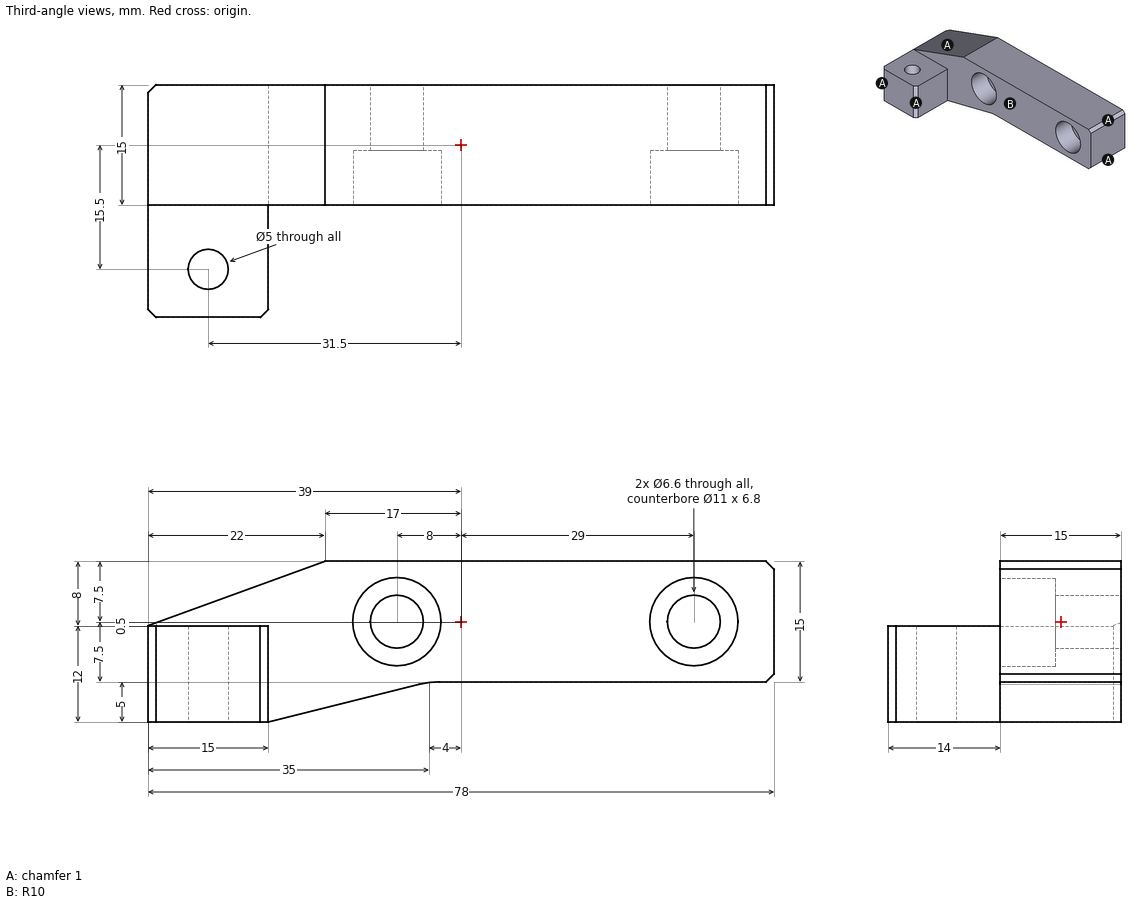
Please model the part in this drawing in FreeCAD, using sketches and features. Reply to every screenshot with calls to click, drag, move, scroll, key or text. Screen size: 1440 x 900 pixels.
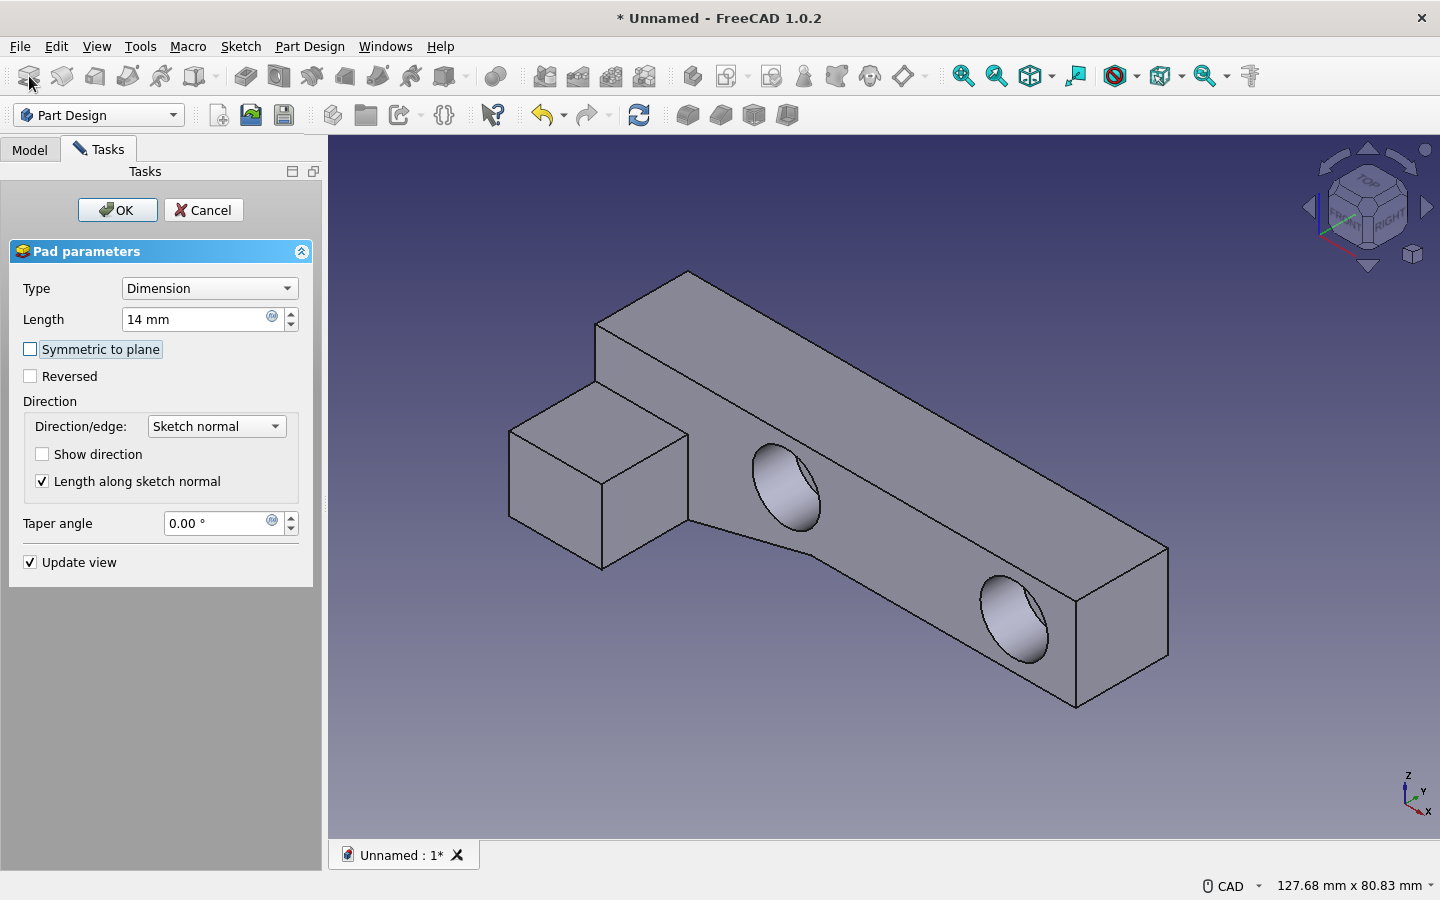
click(118, 210)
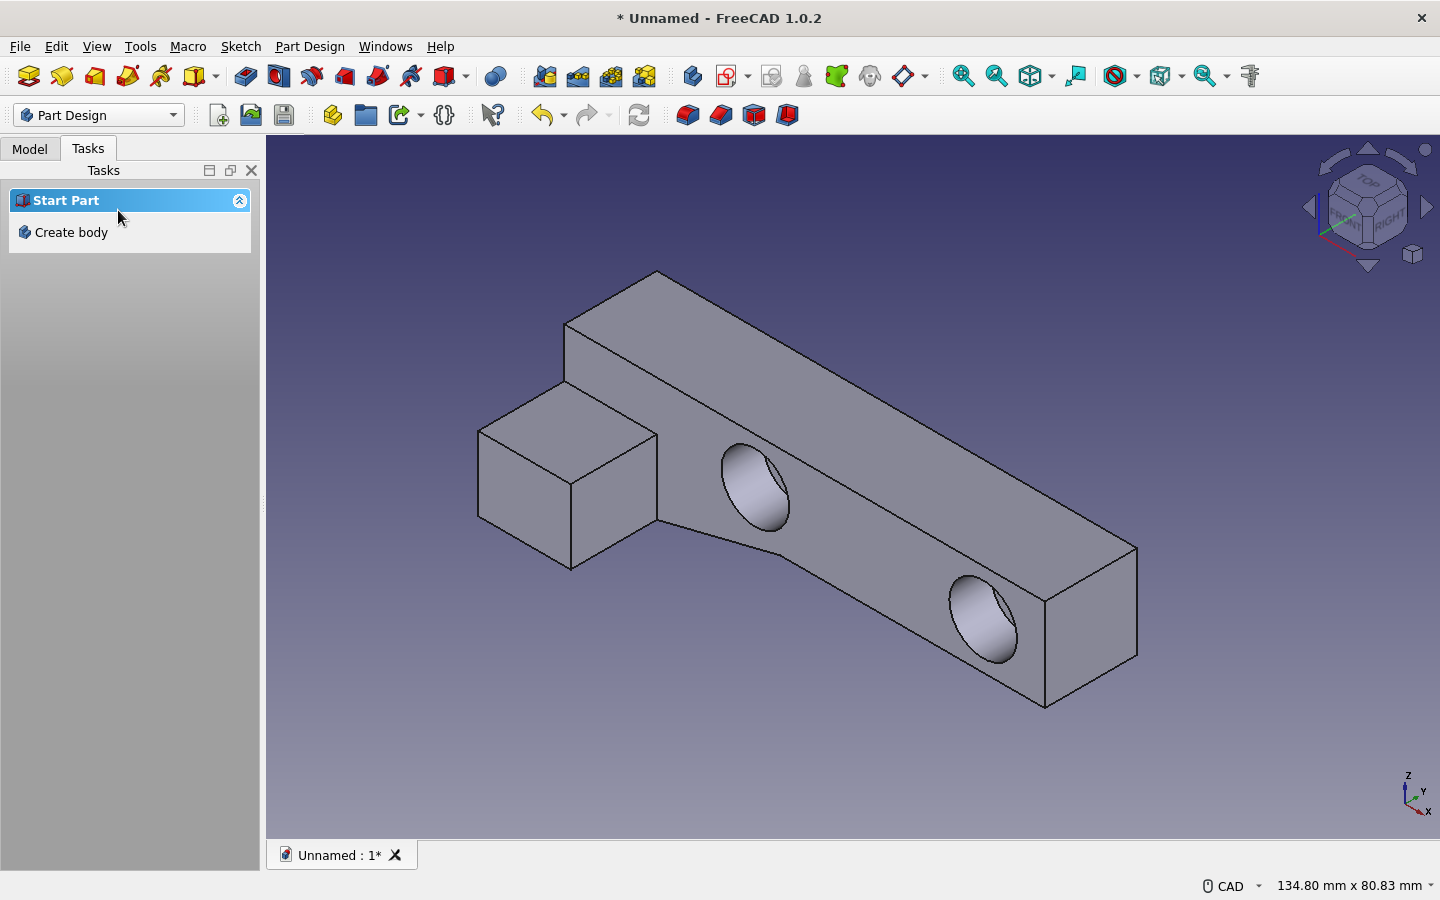
click(568, 432)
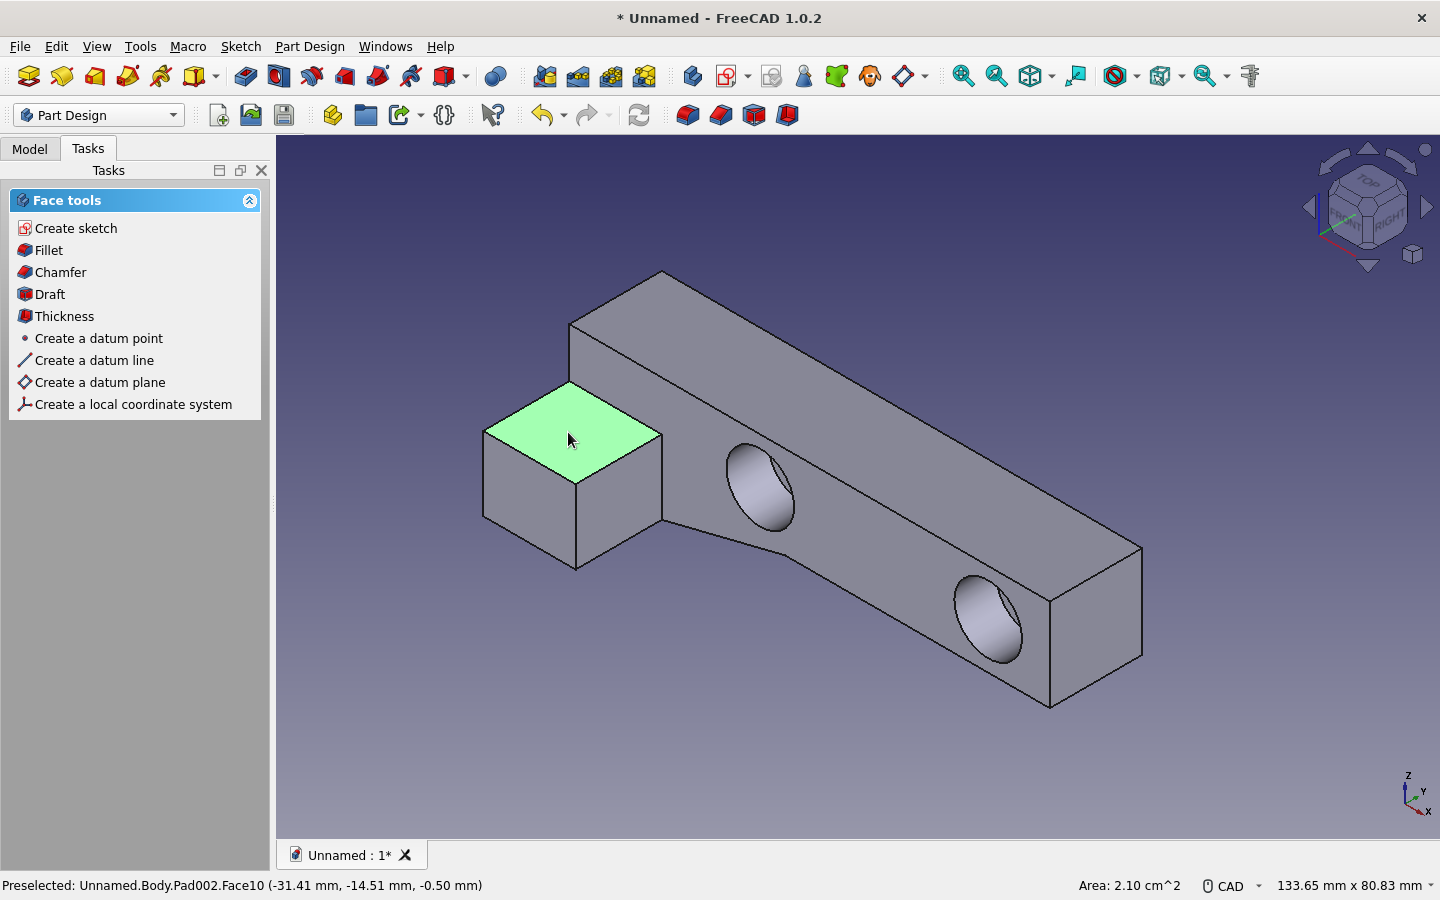
click(726, 76)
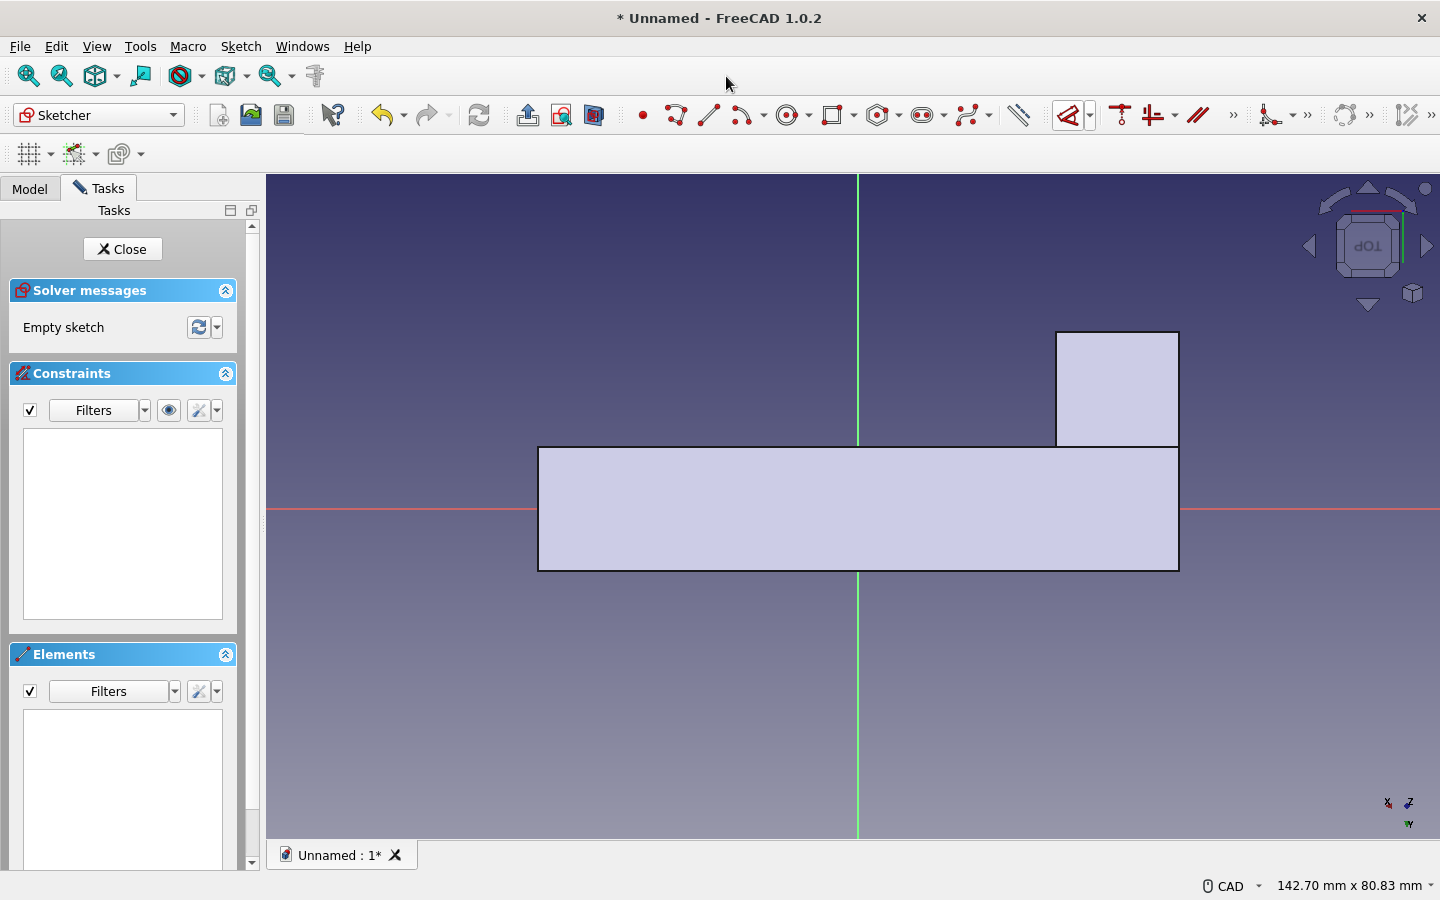
key(q)
key(s)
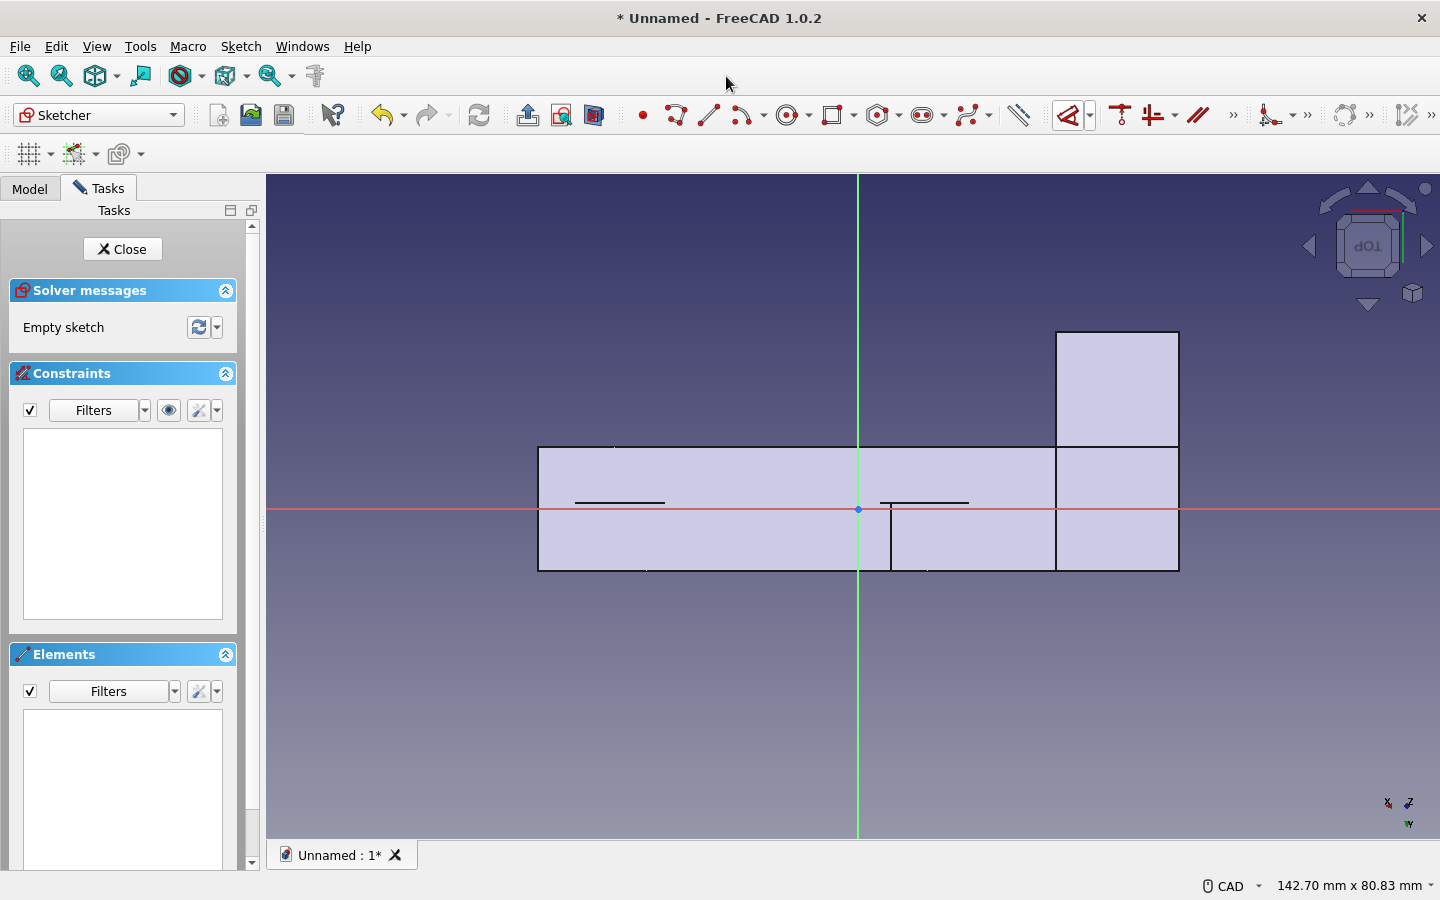
scroll(1151, 369, up, 12)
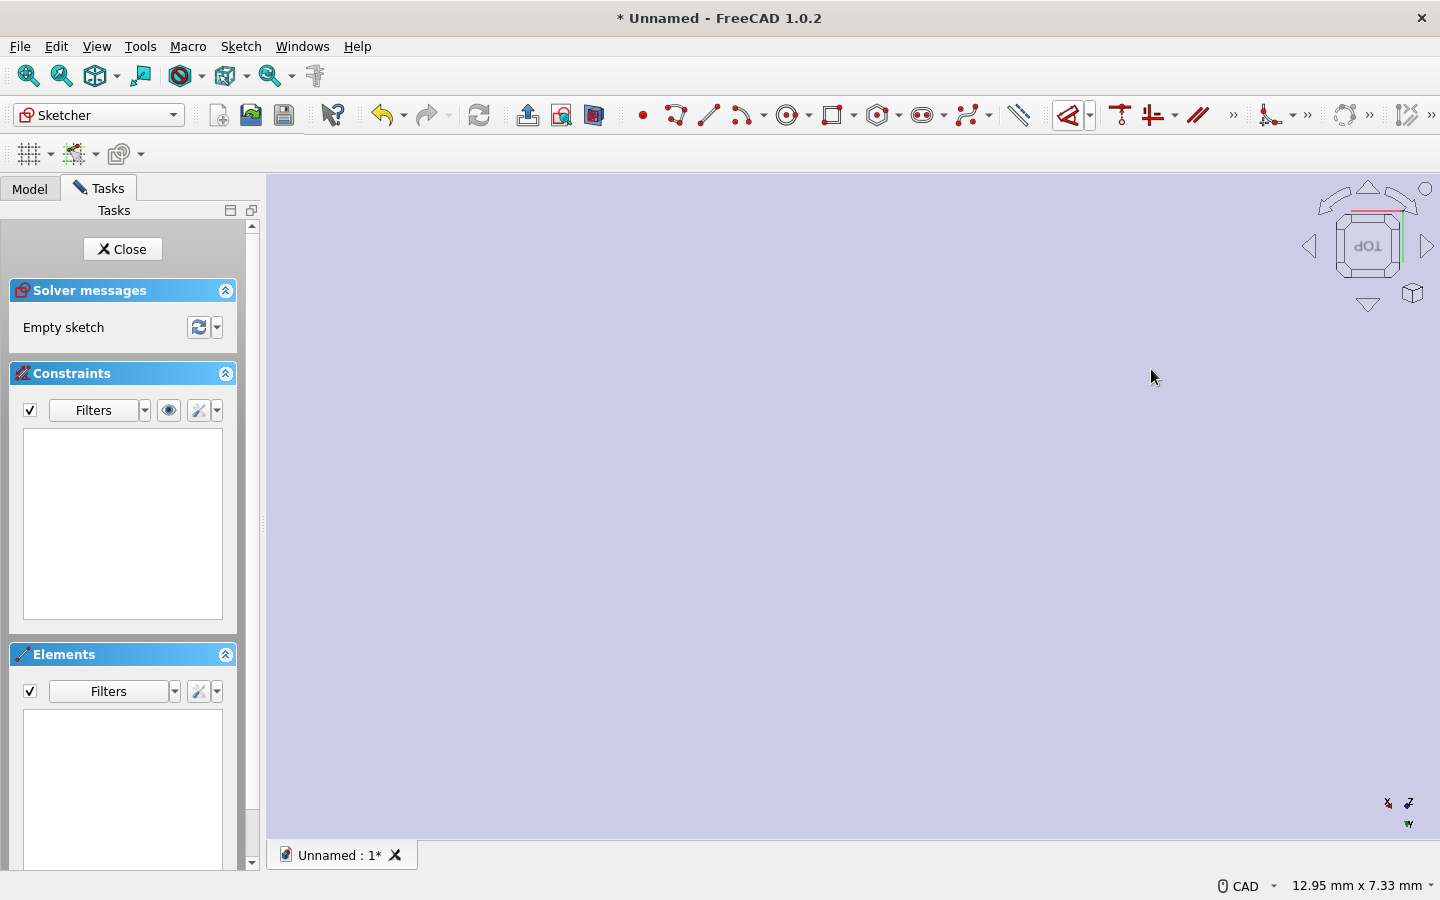
click(786, 116)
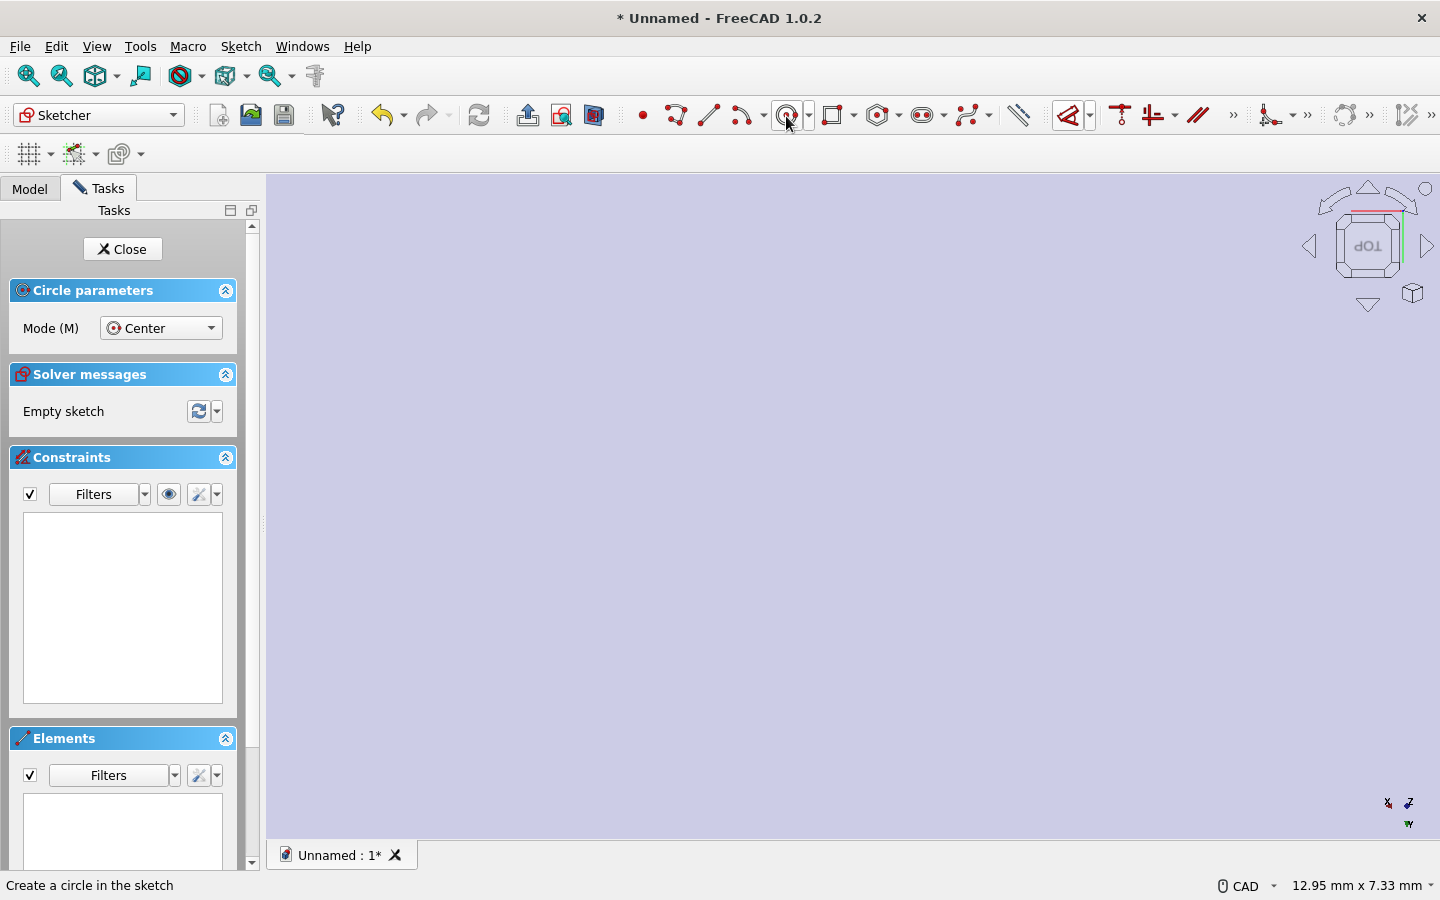
click(775, 504)
move(936, 343)